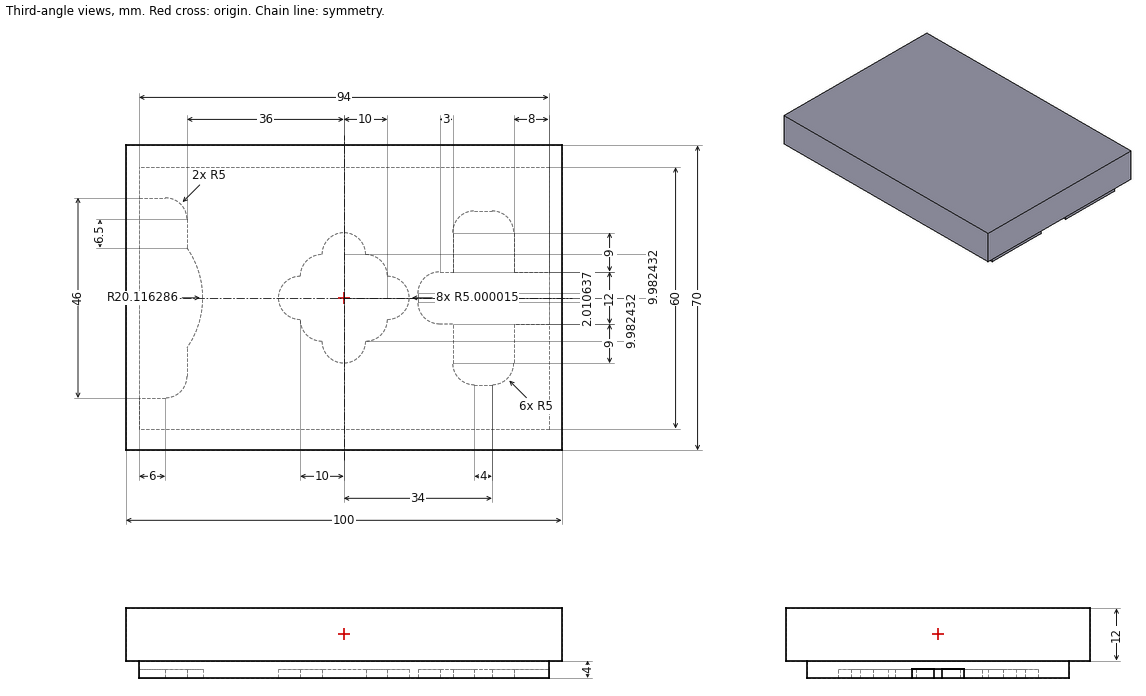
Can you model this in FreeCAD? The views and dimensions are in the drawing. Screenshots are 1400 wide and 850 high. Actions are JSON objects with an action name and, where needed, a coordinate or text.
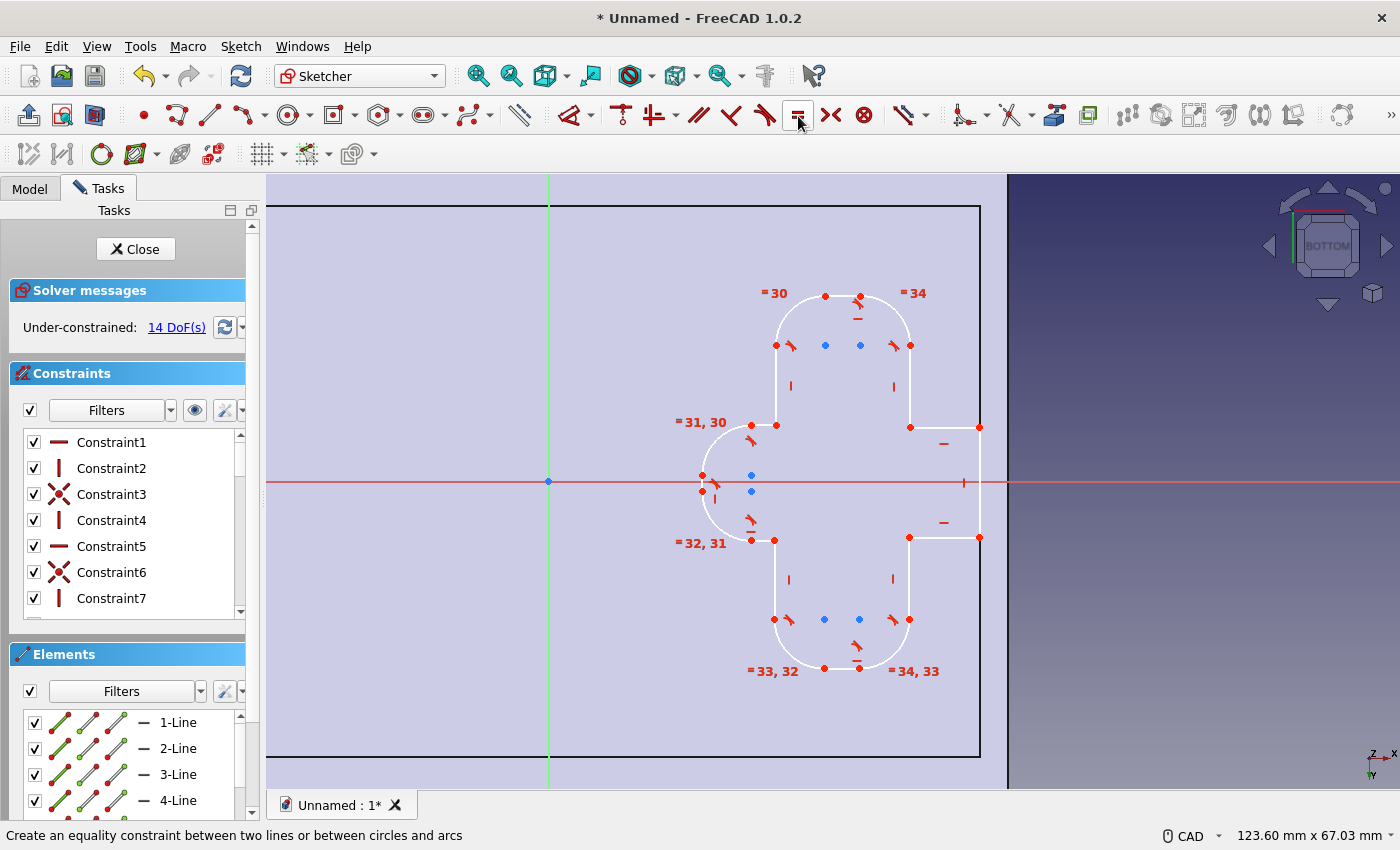
{"action": "left_click", "coordinate": [826, 346]}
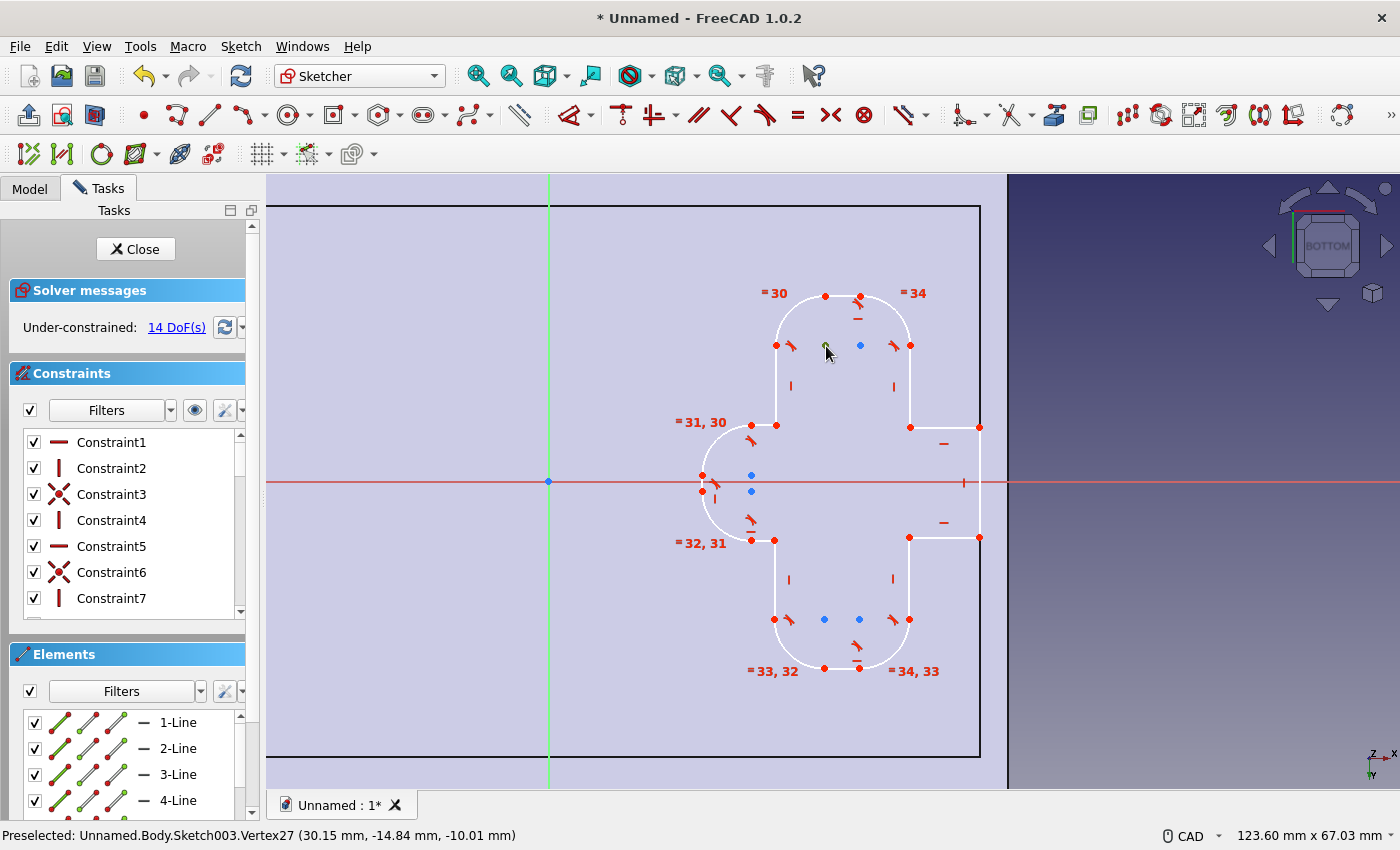
{"action": "left_click", "coordinate": [824, 619]}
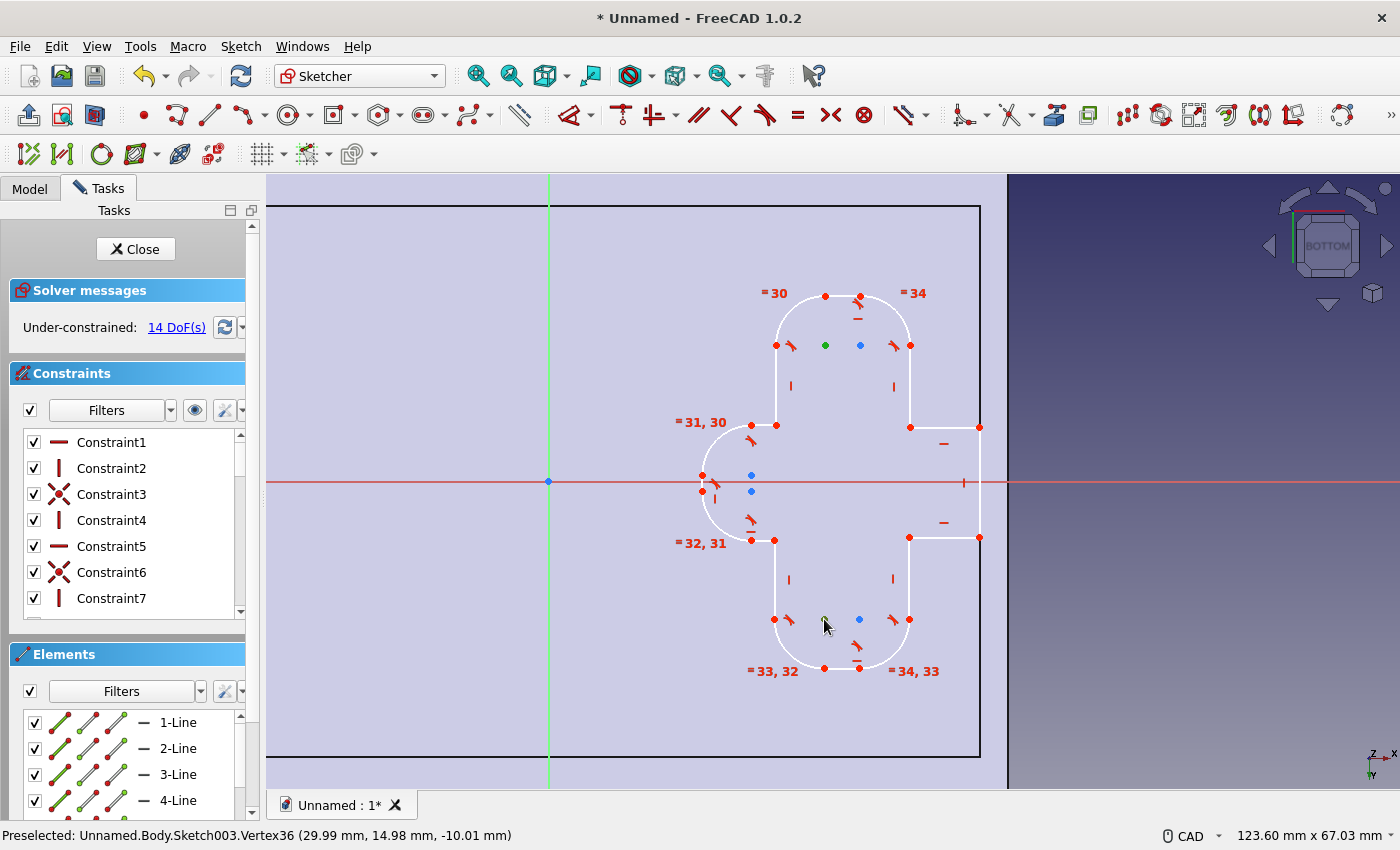
{"action": "left_click", "coordinate": [361, 482]}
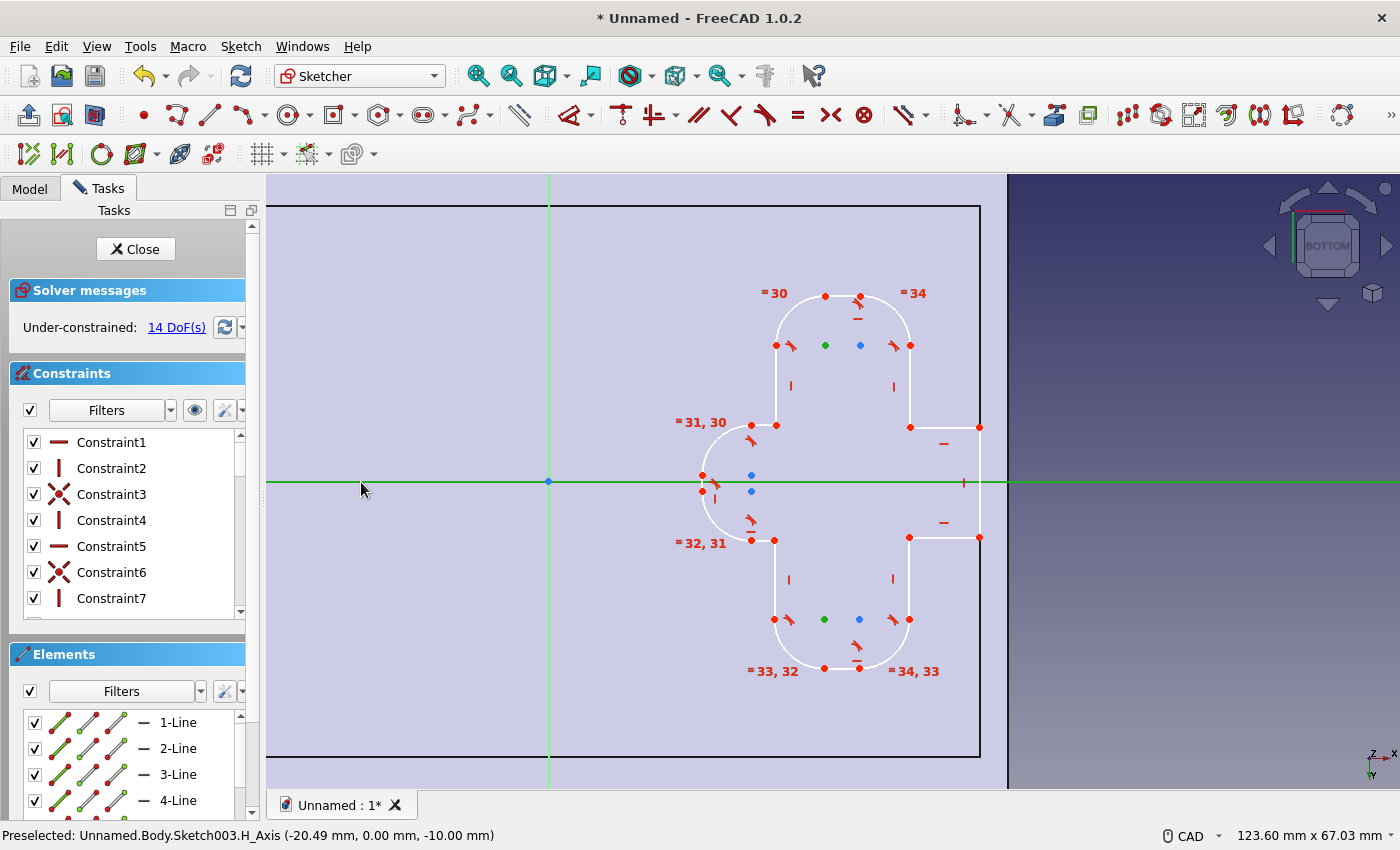
{"action": "left_click", "coordinate": [831, 116]}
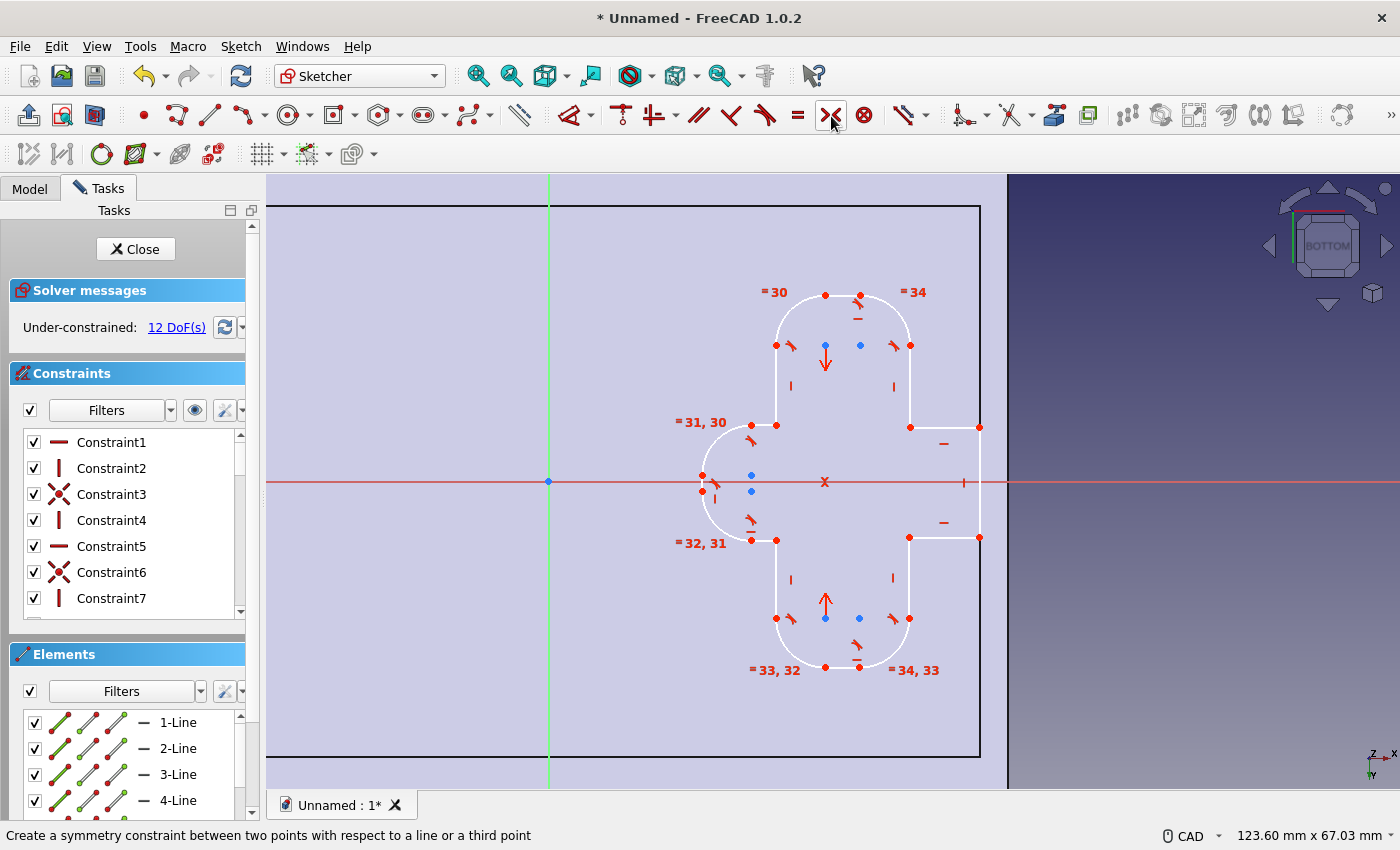
{"action": "left_click", "coordinate": [909, 538]}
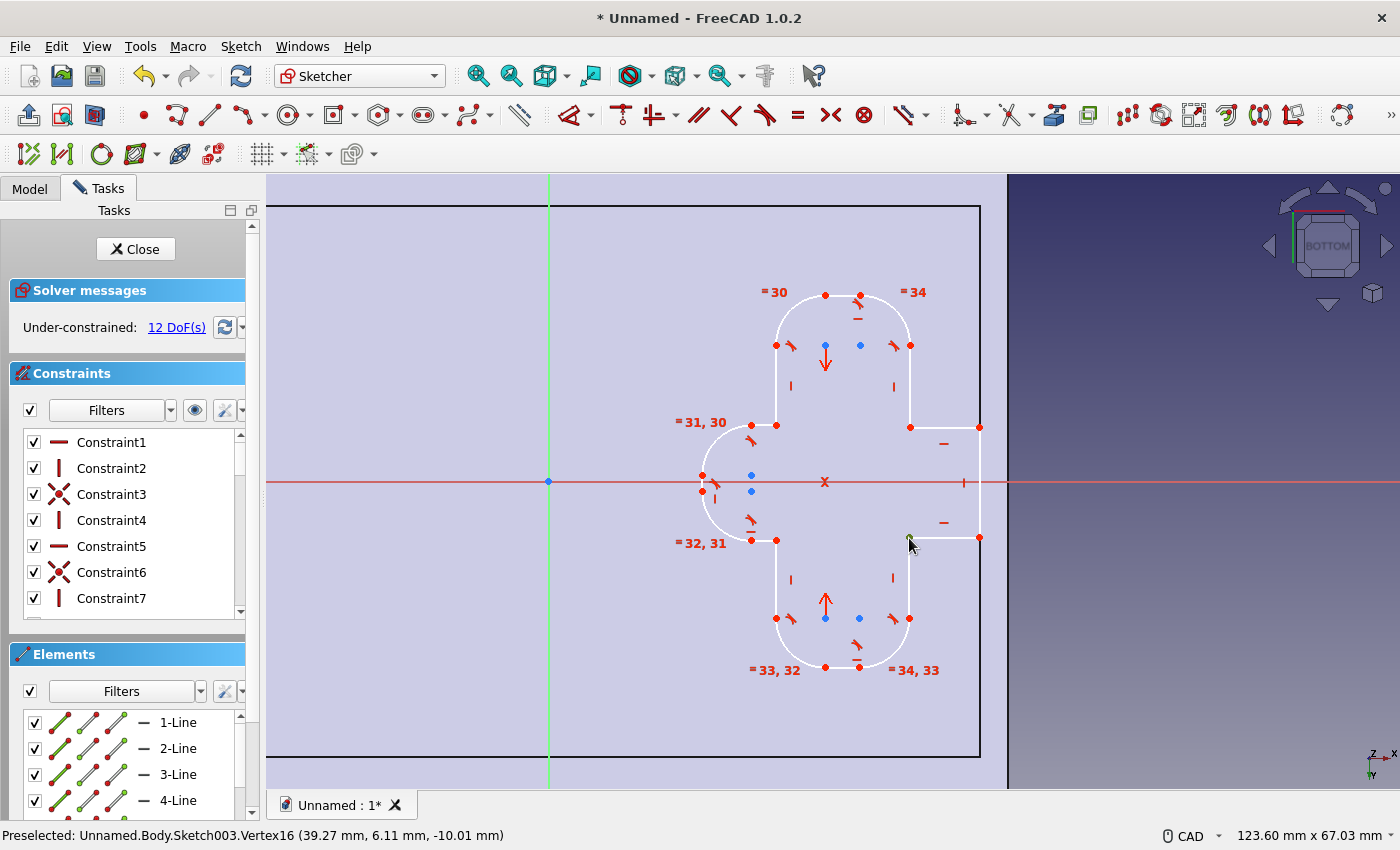
{"action": "left_click", "coordinate": [910, 428]}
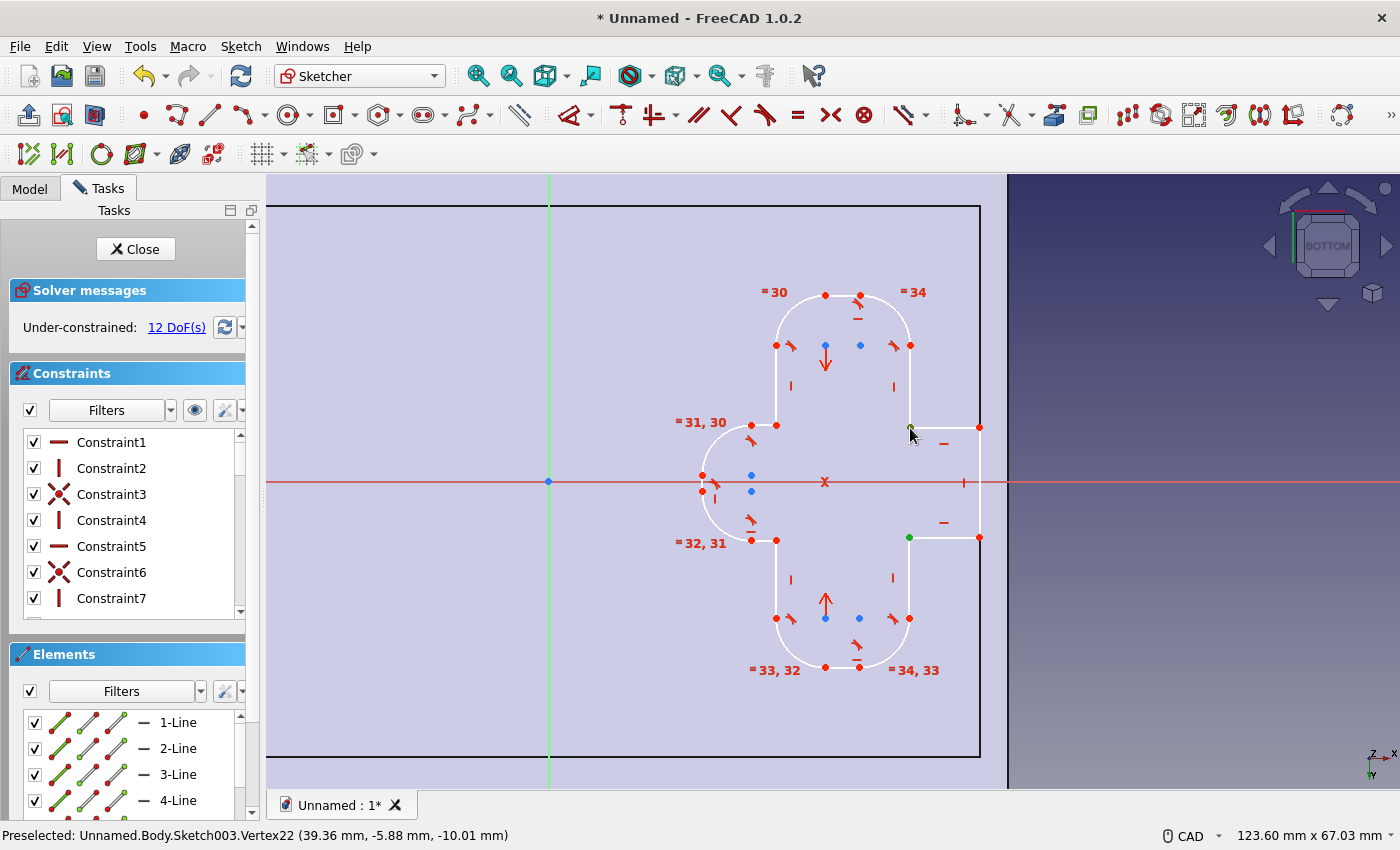
{"action": "left_click", "coordinate": [361, 482]}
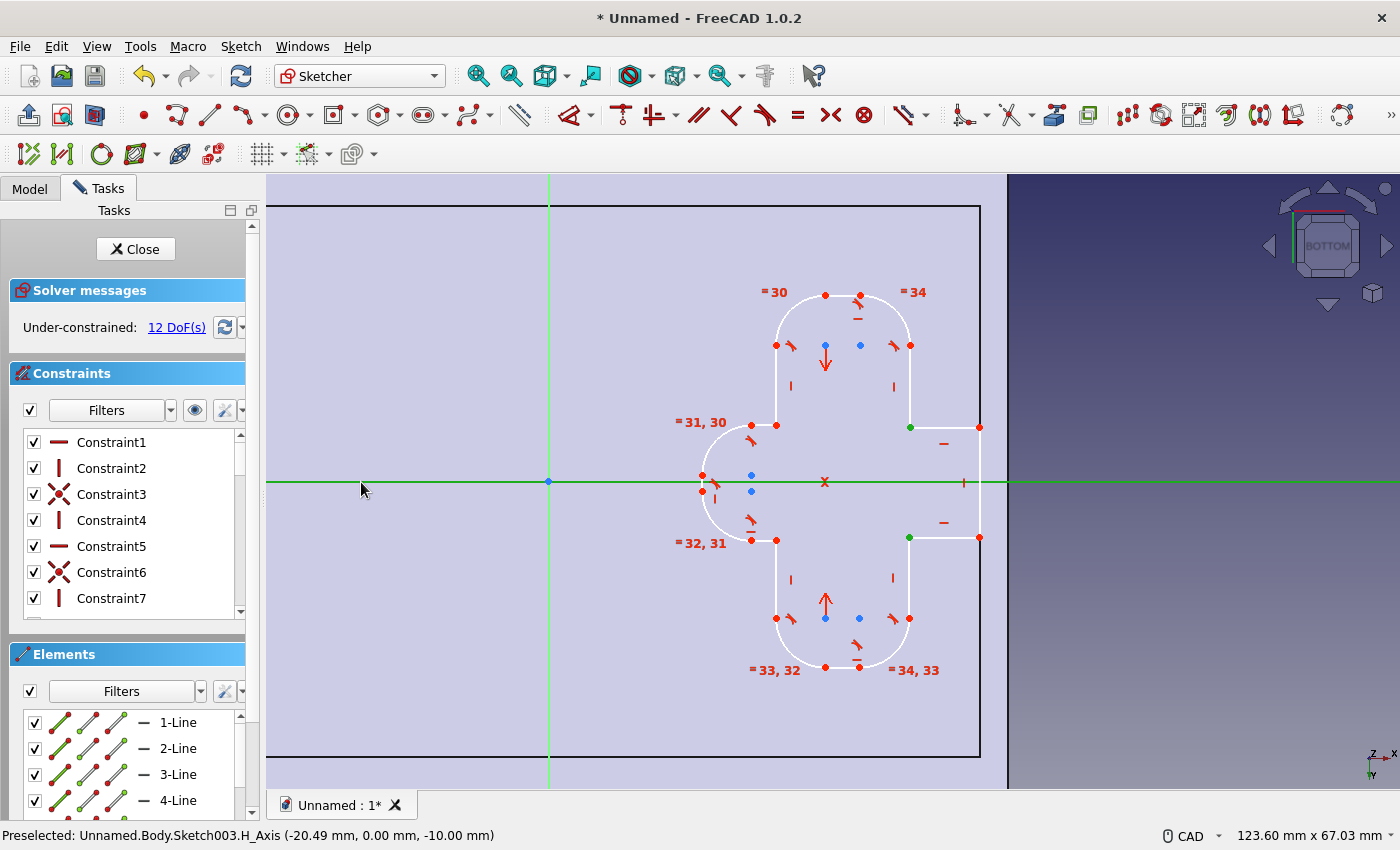
{"action": "left_click", "coordinate": [831, 116]}